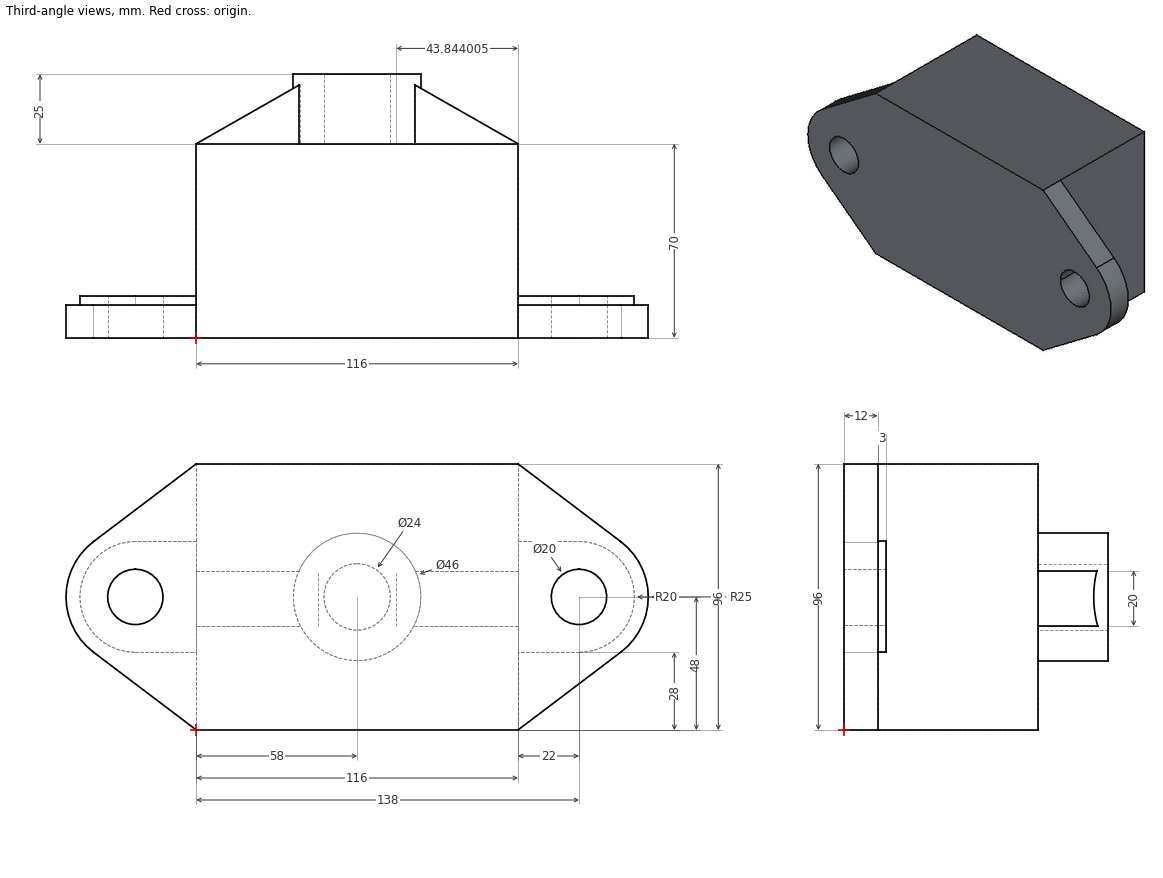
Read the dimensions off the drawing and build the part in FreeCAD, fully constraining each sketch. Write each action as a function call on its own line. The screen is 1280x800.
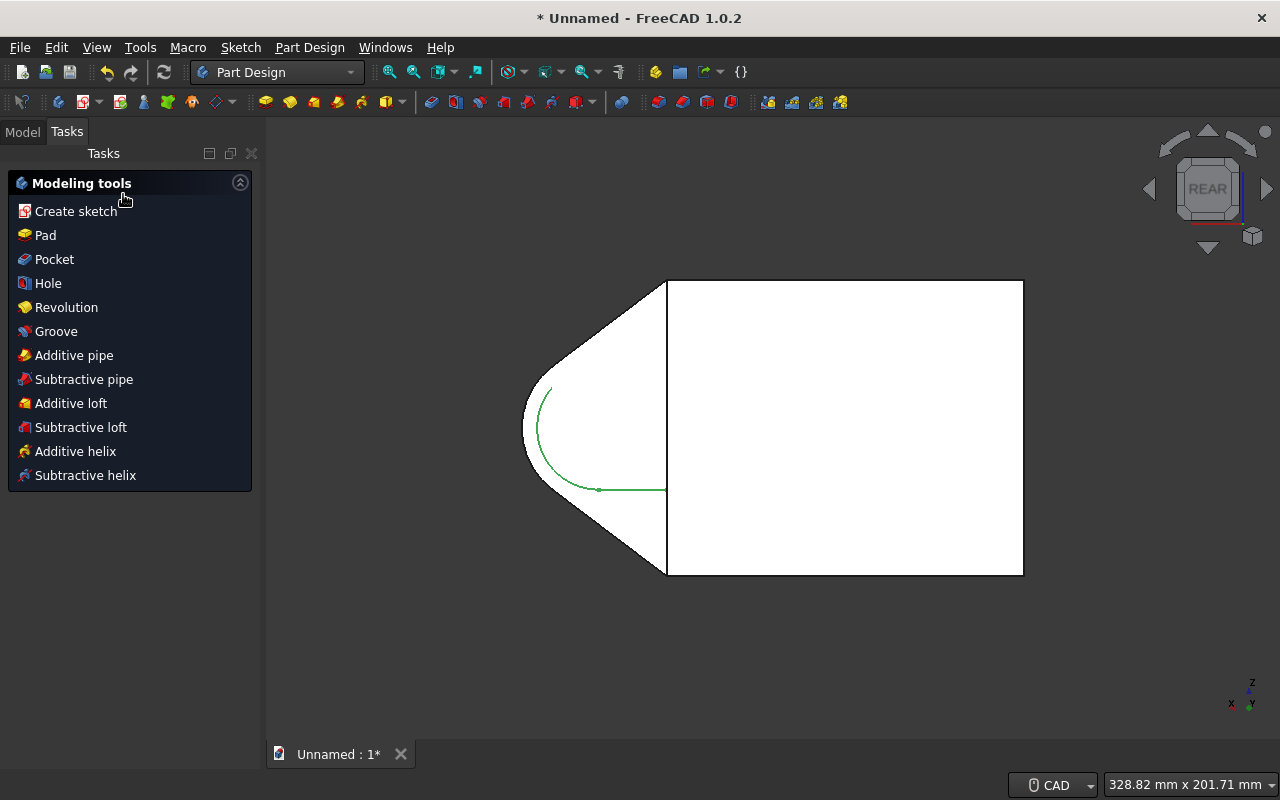
click(266, 102)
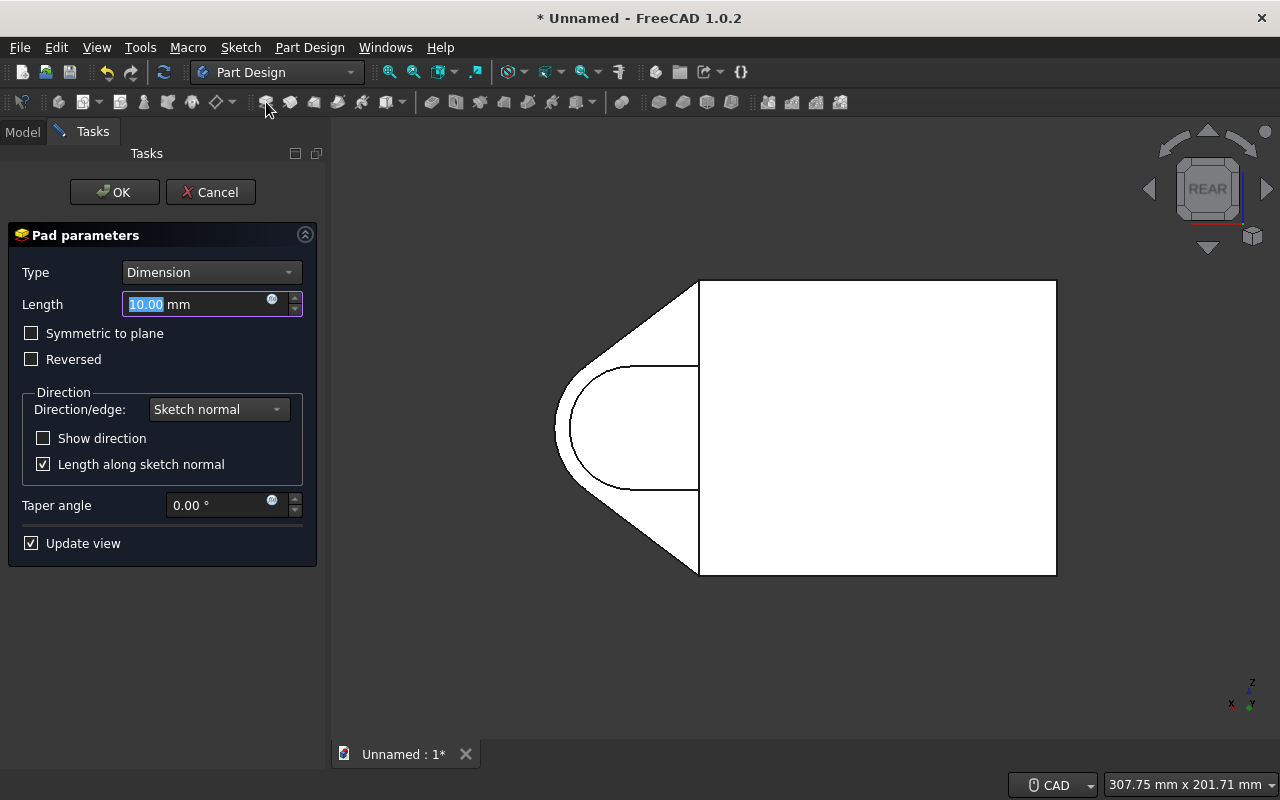
text(3)
key(Tab)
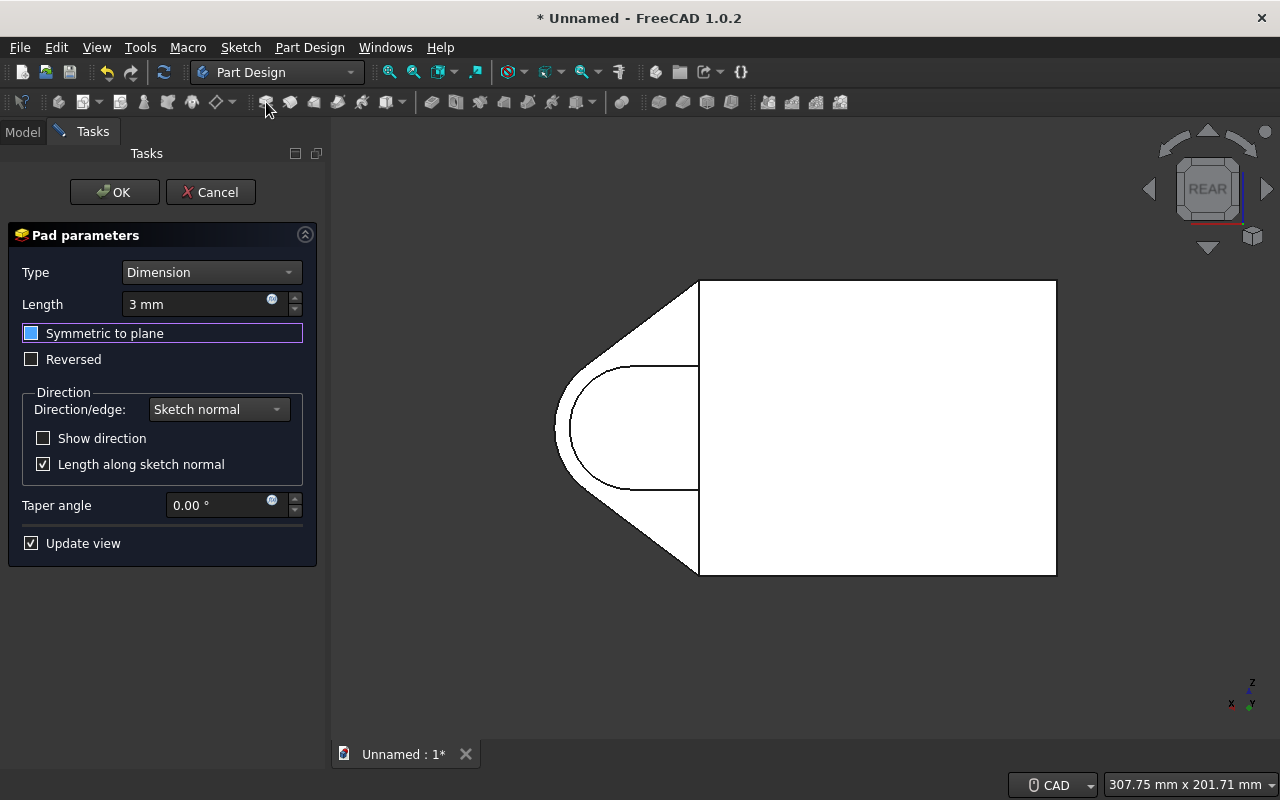
click(115, 192)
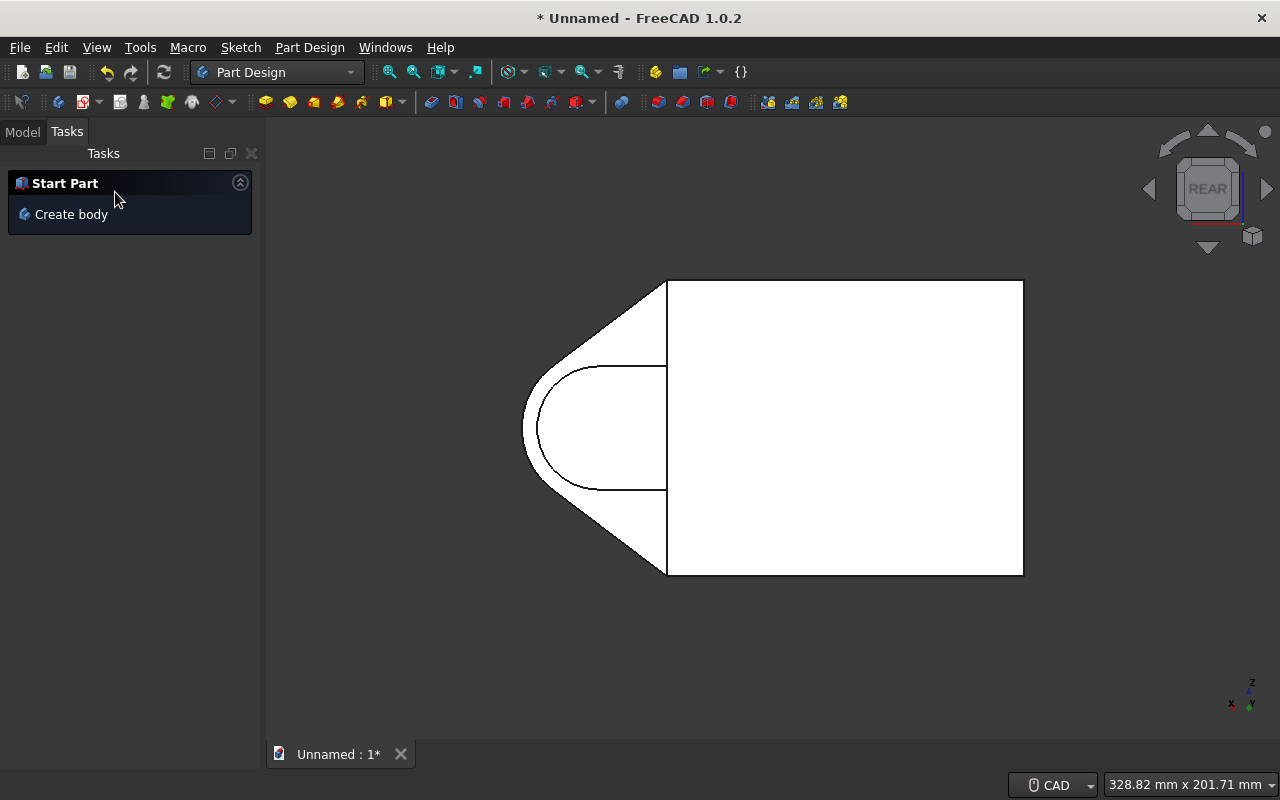
click(602, 427)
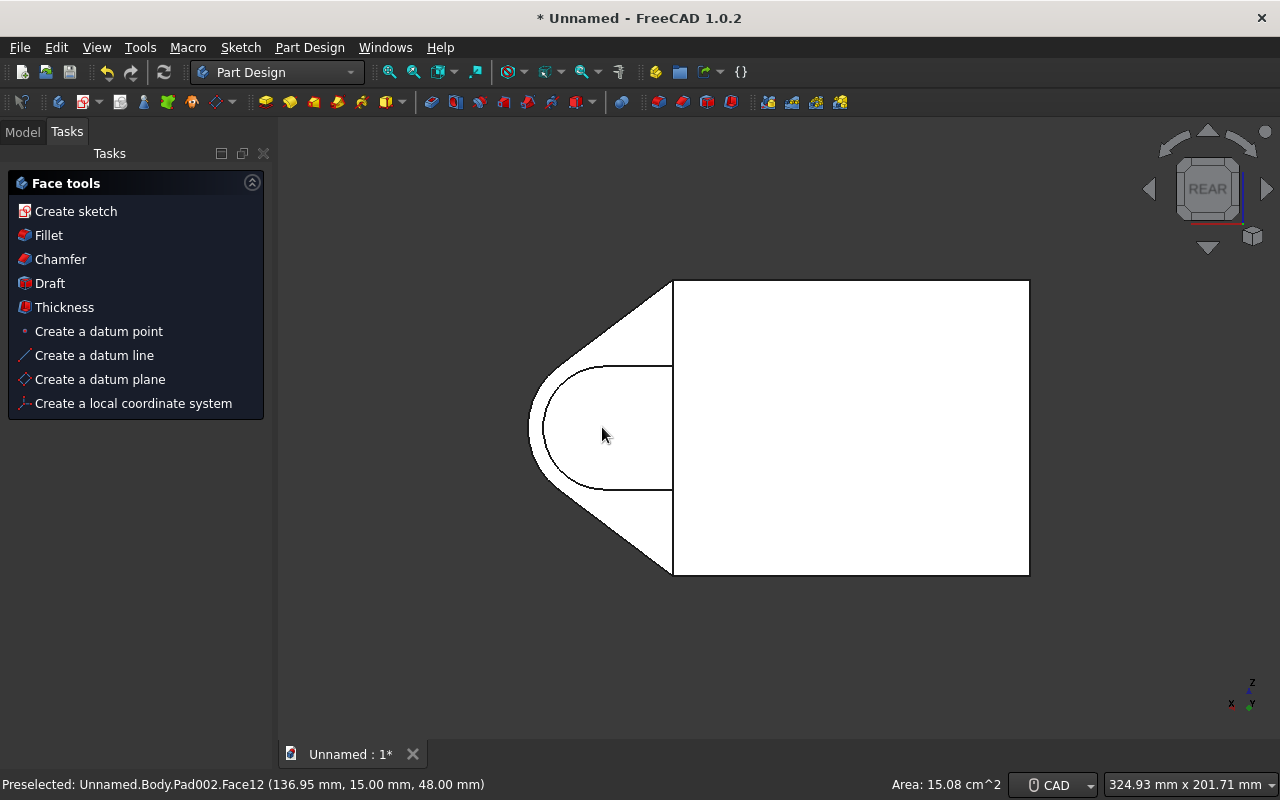
click(84, 102)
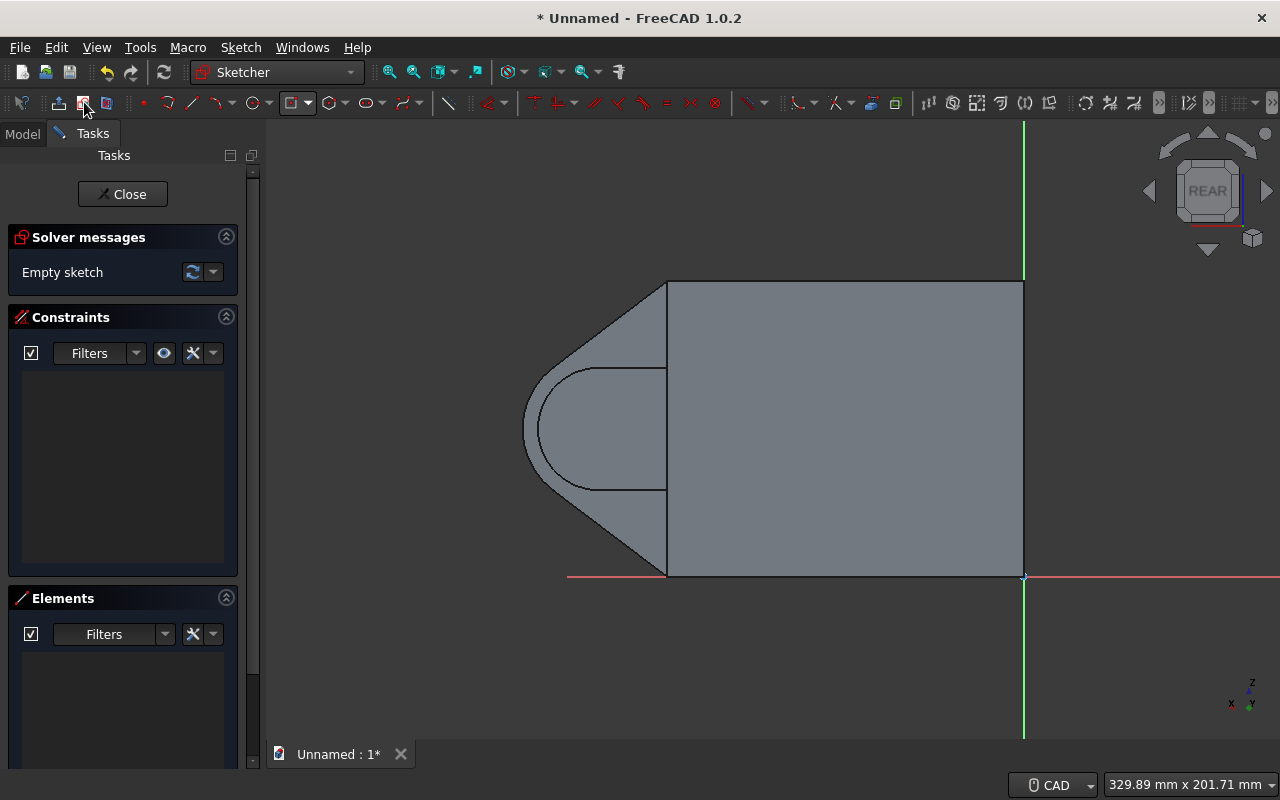
scroll(579, 429, up, 9)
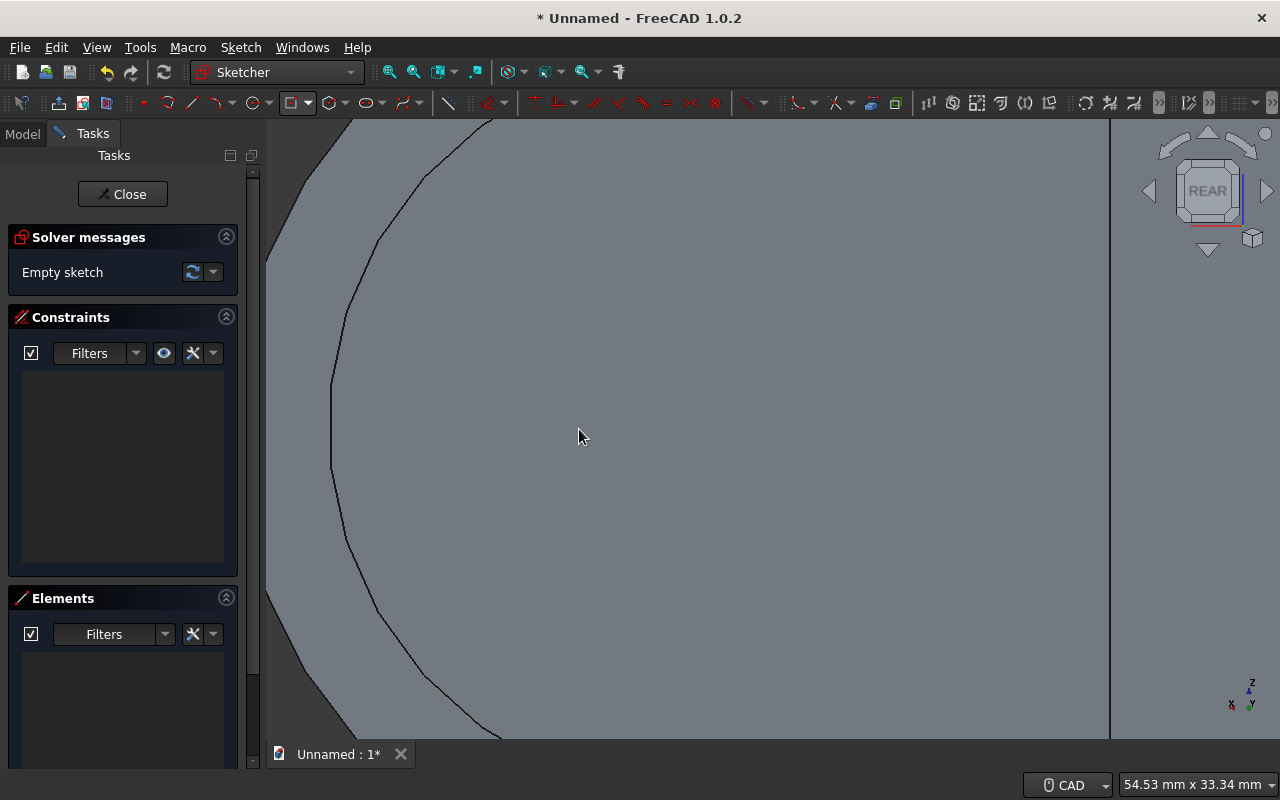
click(254, 104)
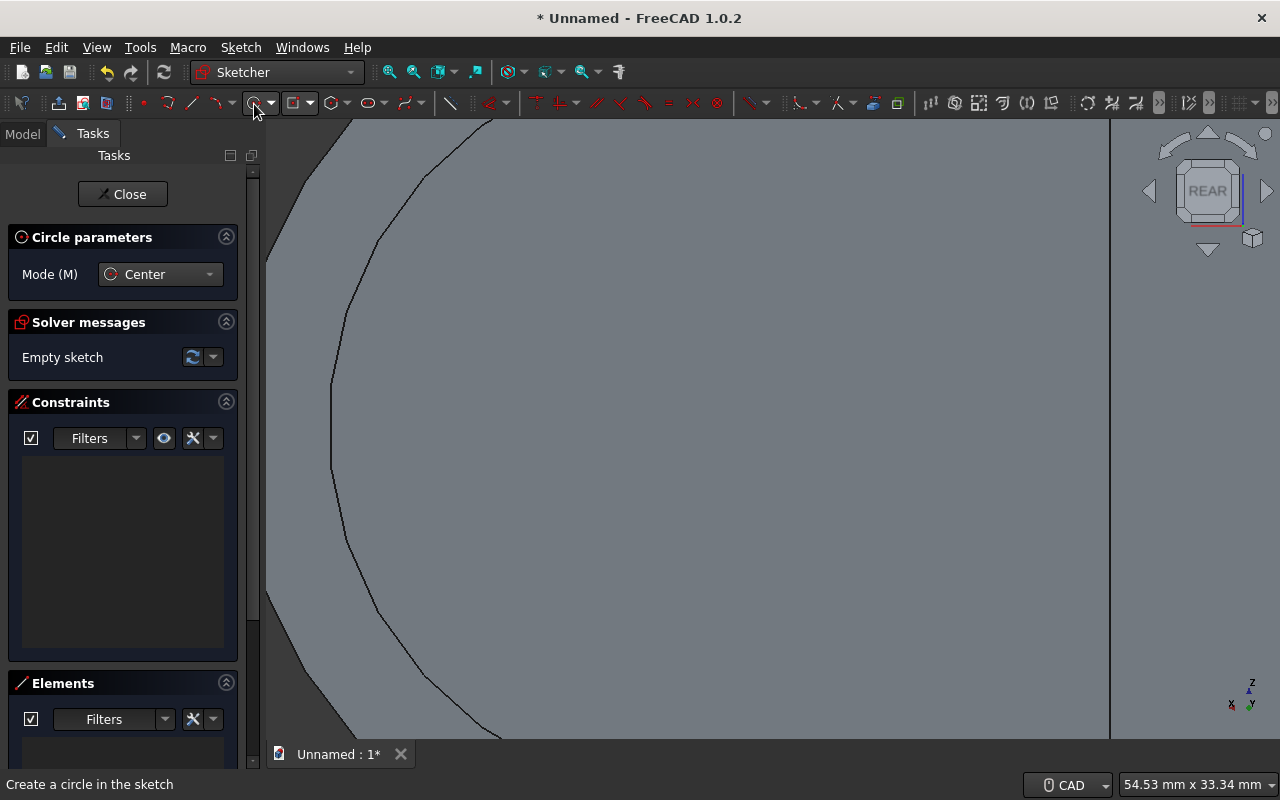
click(700, 426)
move(832, 295)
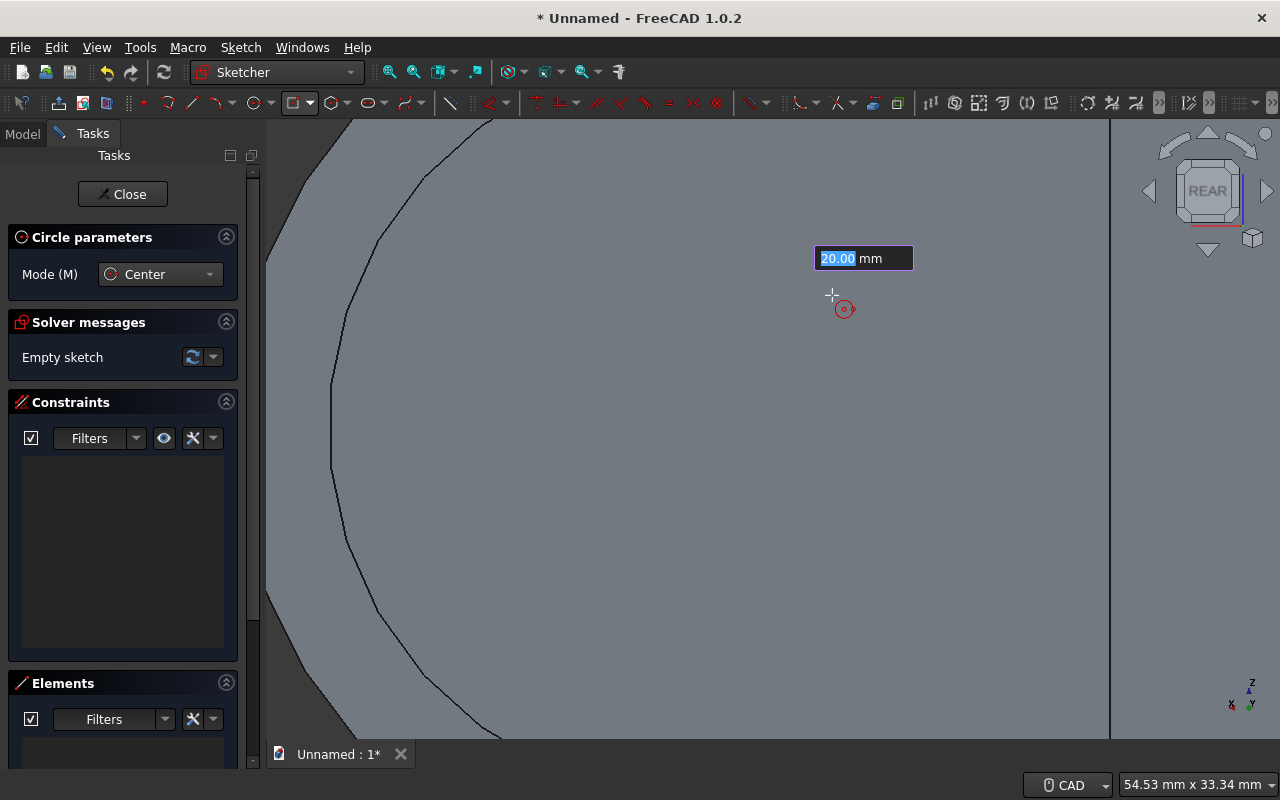
text(20)
key(Return)
key(Escape)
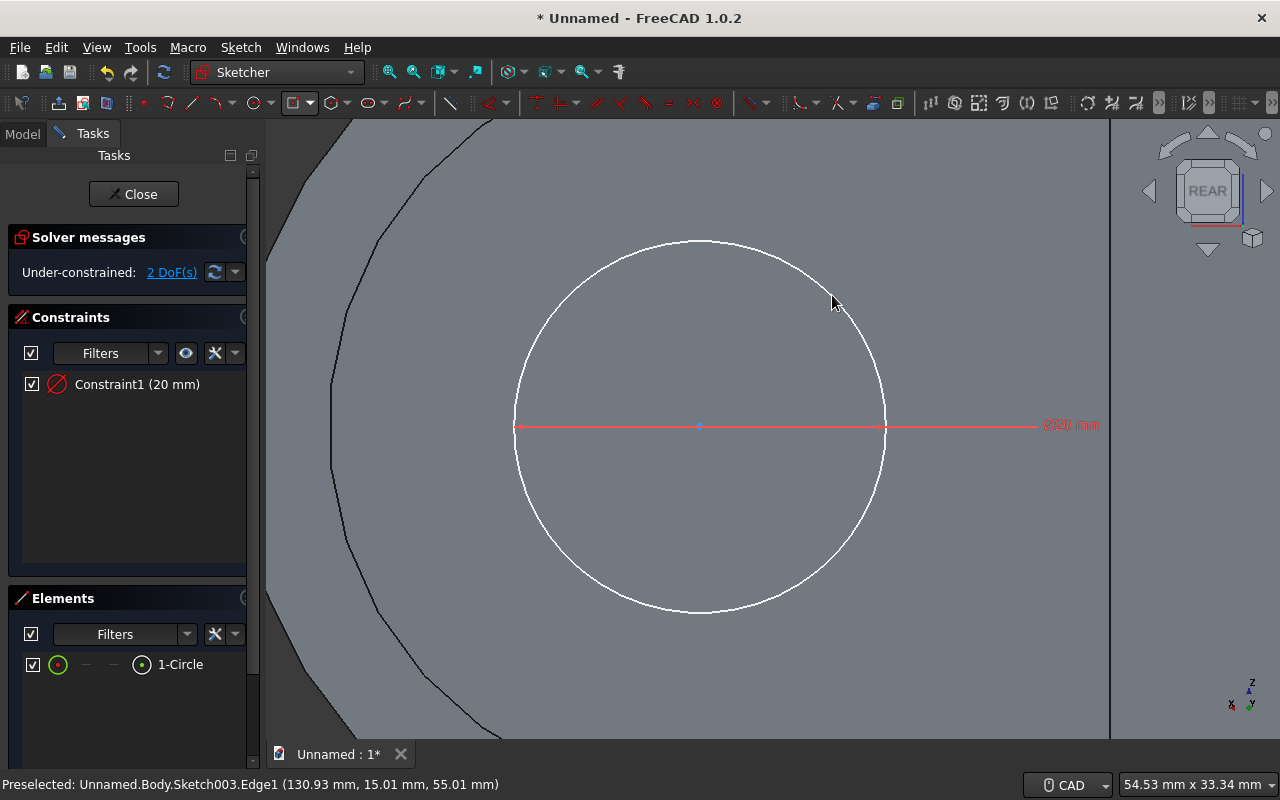
click(490, 104)